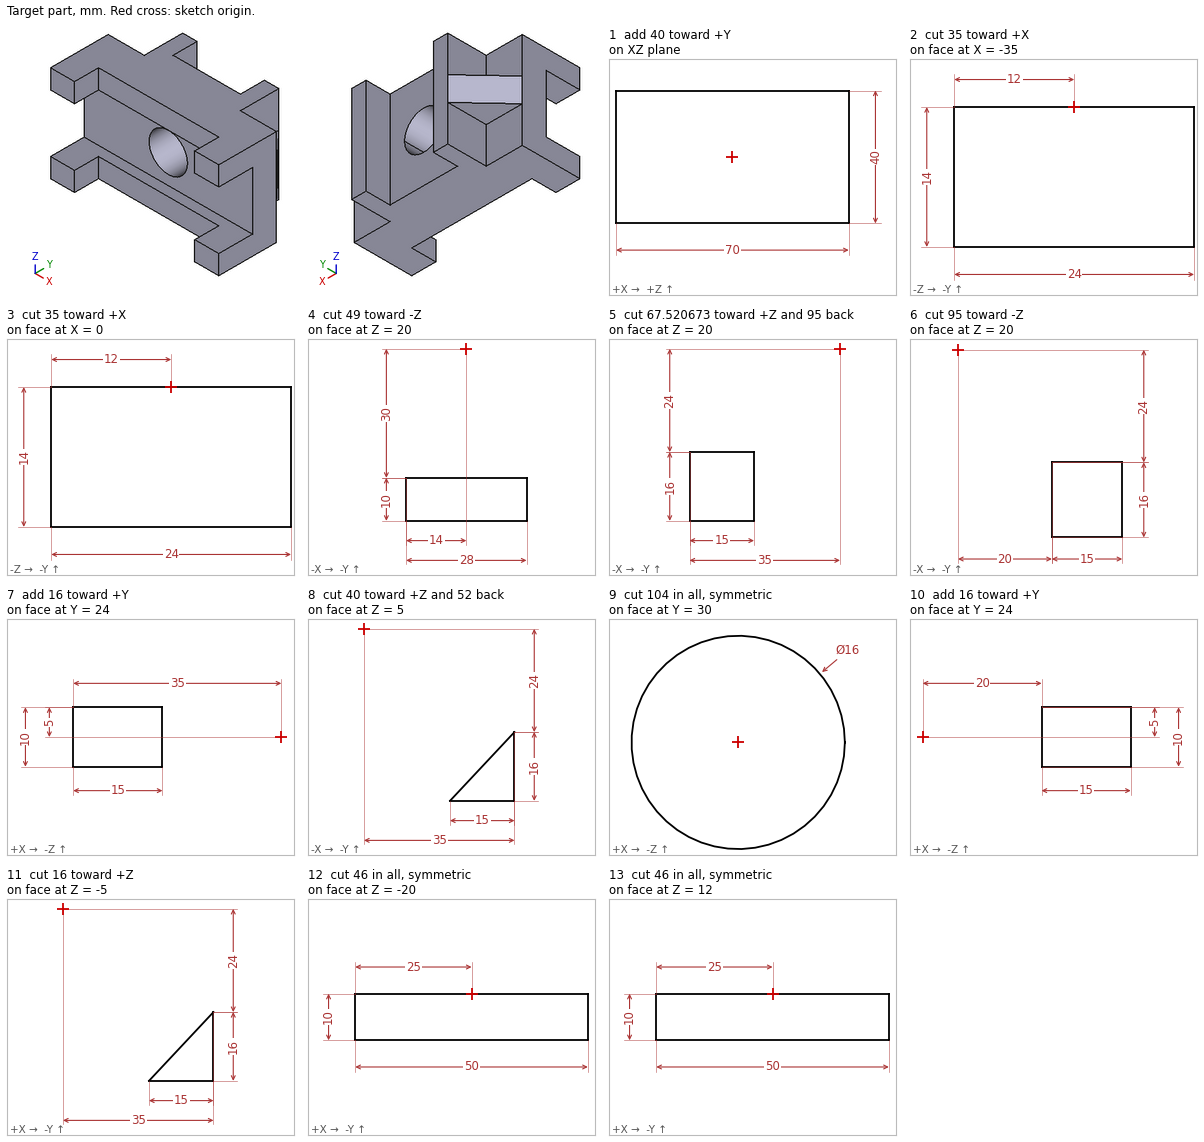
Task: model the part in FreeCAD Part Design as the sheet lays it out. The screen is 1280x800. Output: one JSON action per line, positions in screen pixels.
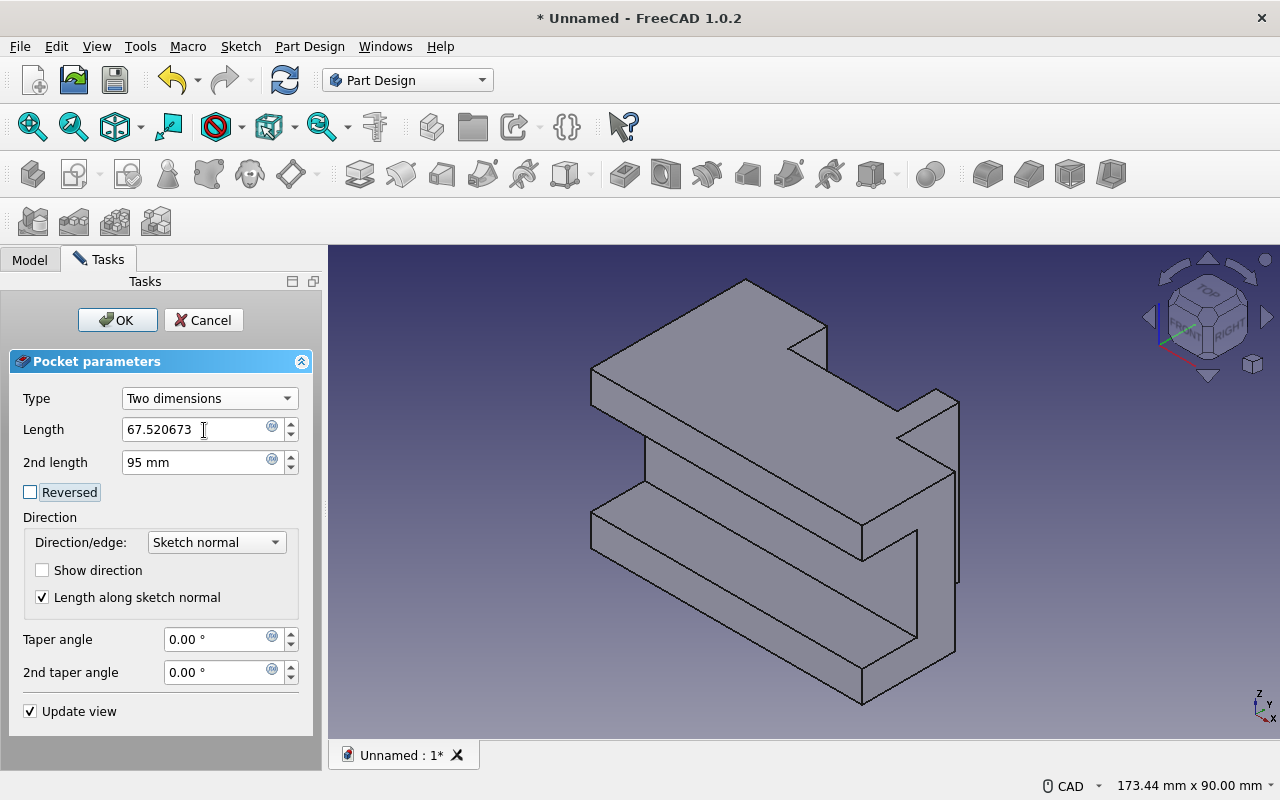
{"action": "left_click", "coordinate": [31, 492]}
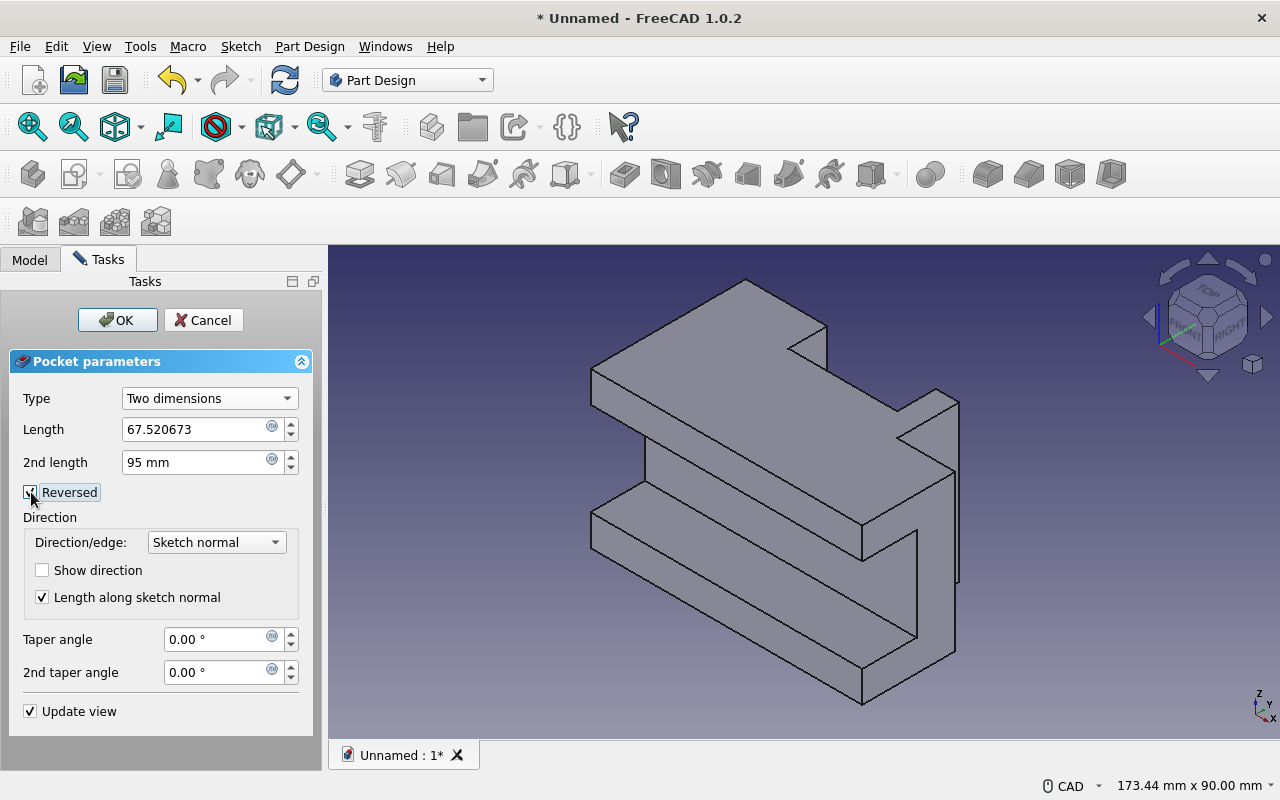
{"action": "left_click", "coordinate": [118, 320]}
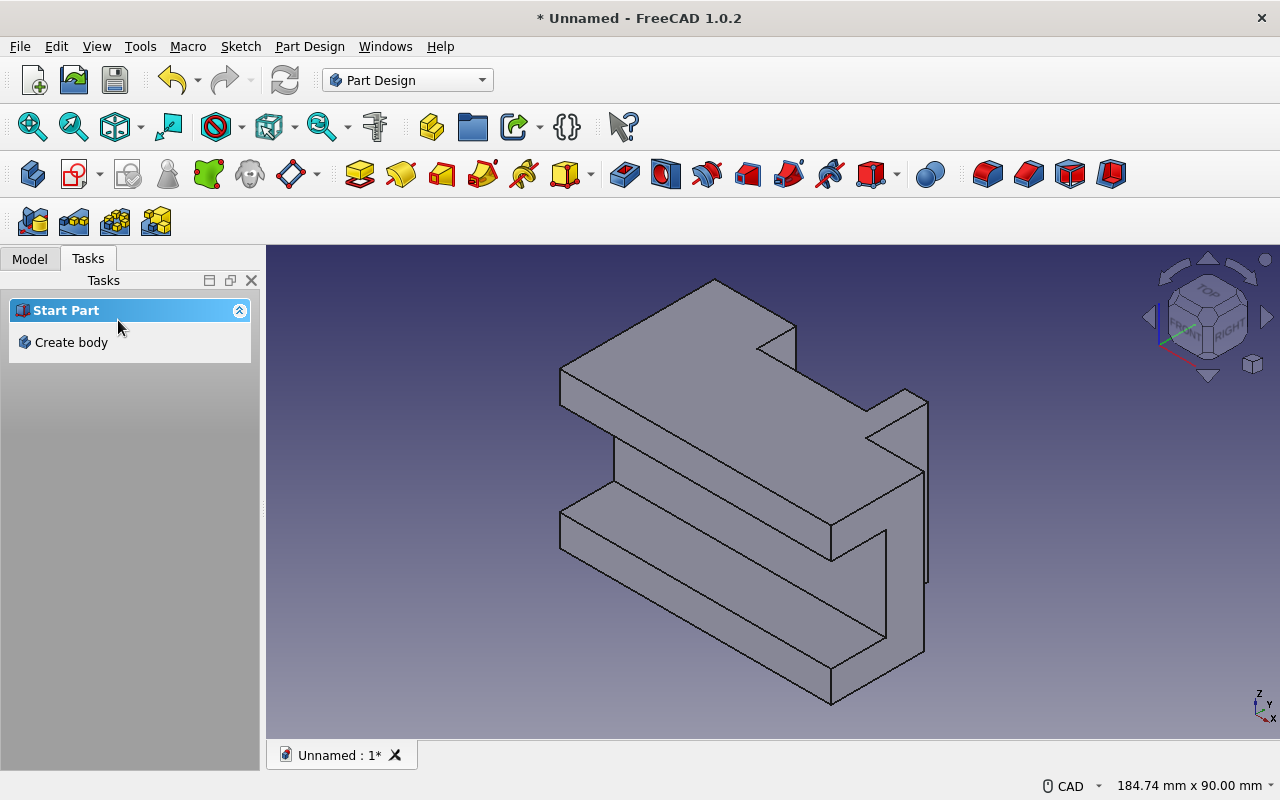
{"action": "left_click", "coordinate": [751, 414]}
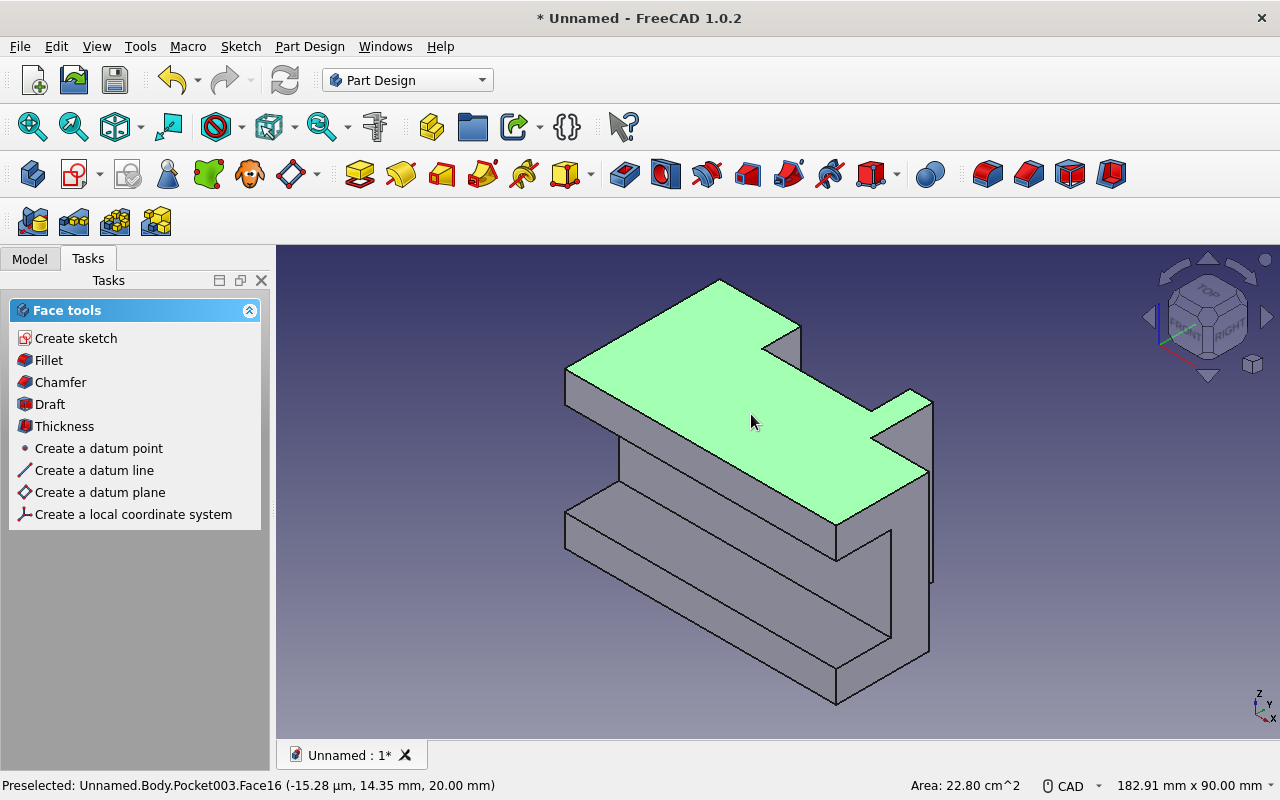
{"action": "left_click", "coordinate": [74, 174]}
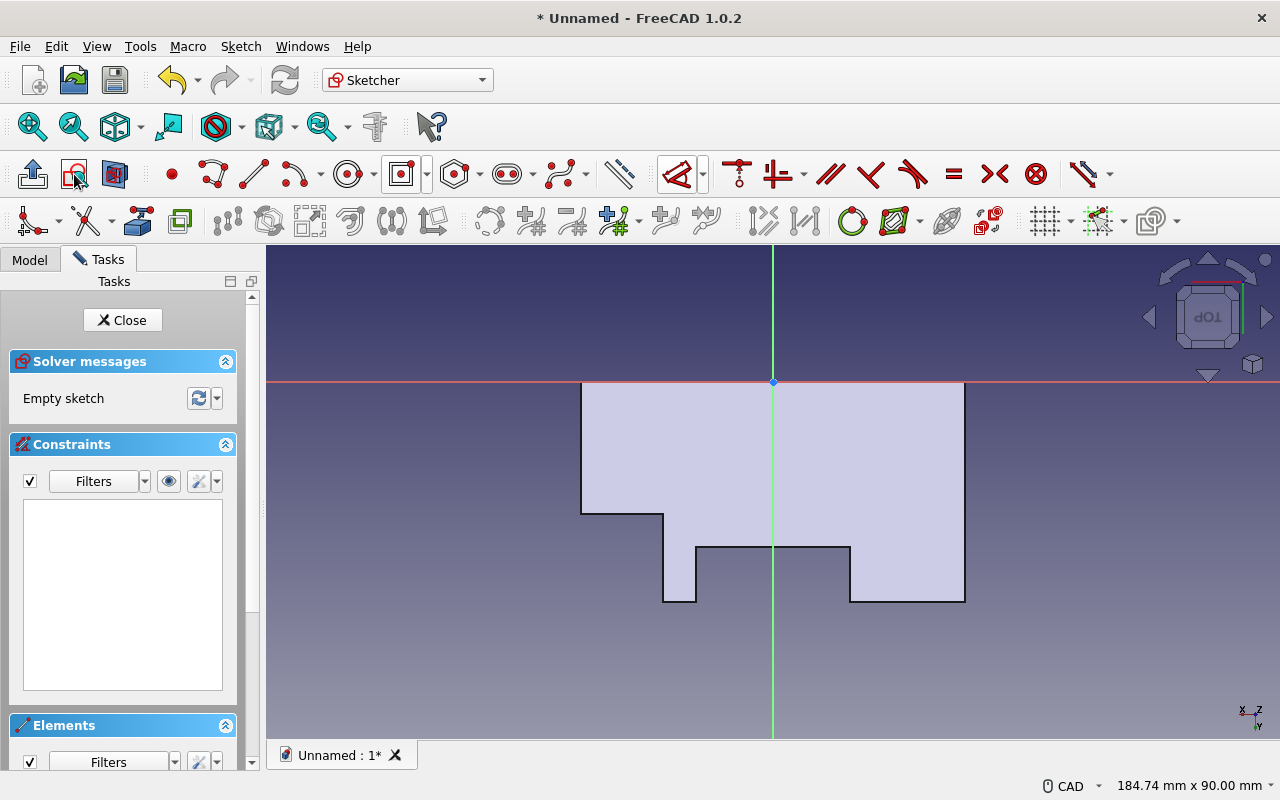
{"action": "scroll", "coordinate": [1019, 586], "scroll_direction": "up", "scroll_amount": 6}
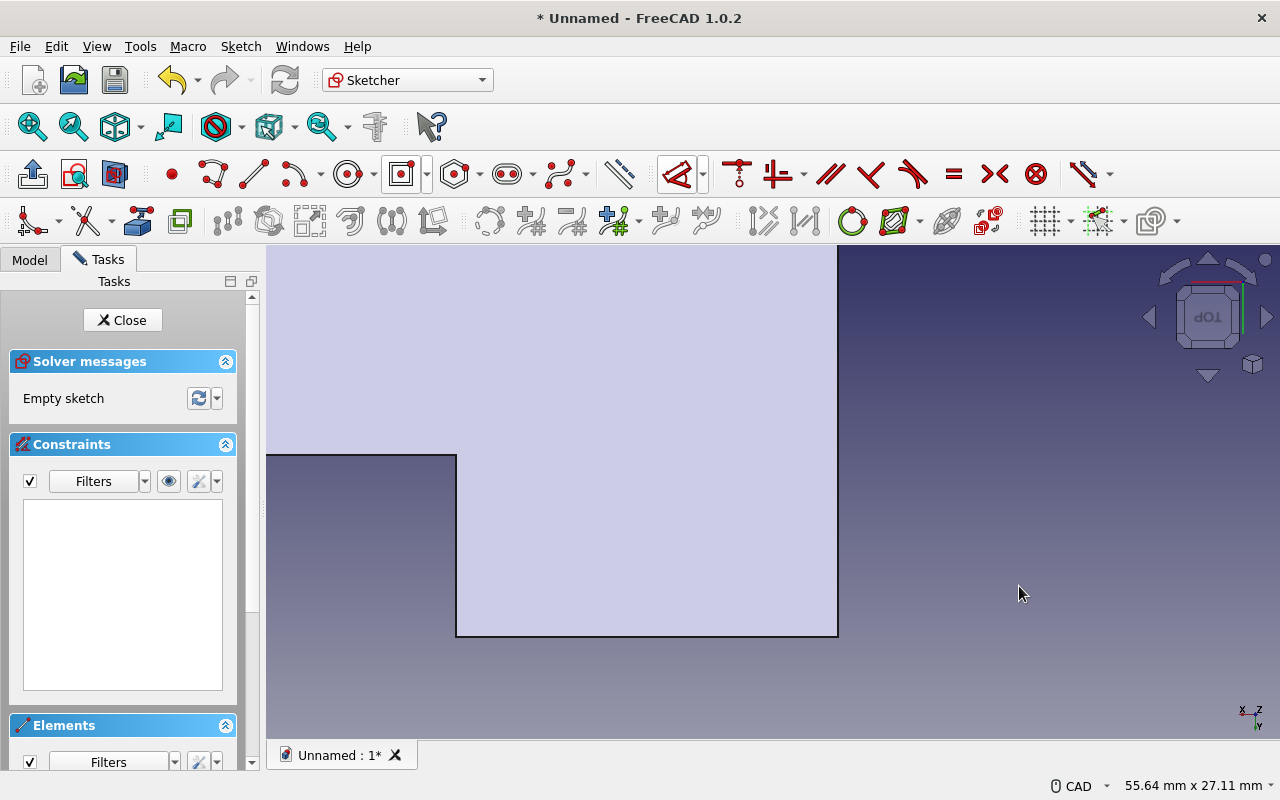
{"action": "key", "text": "g r"}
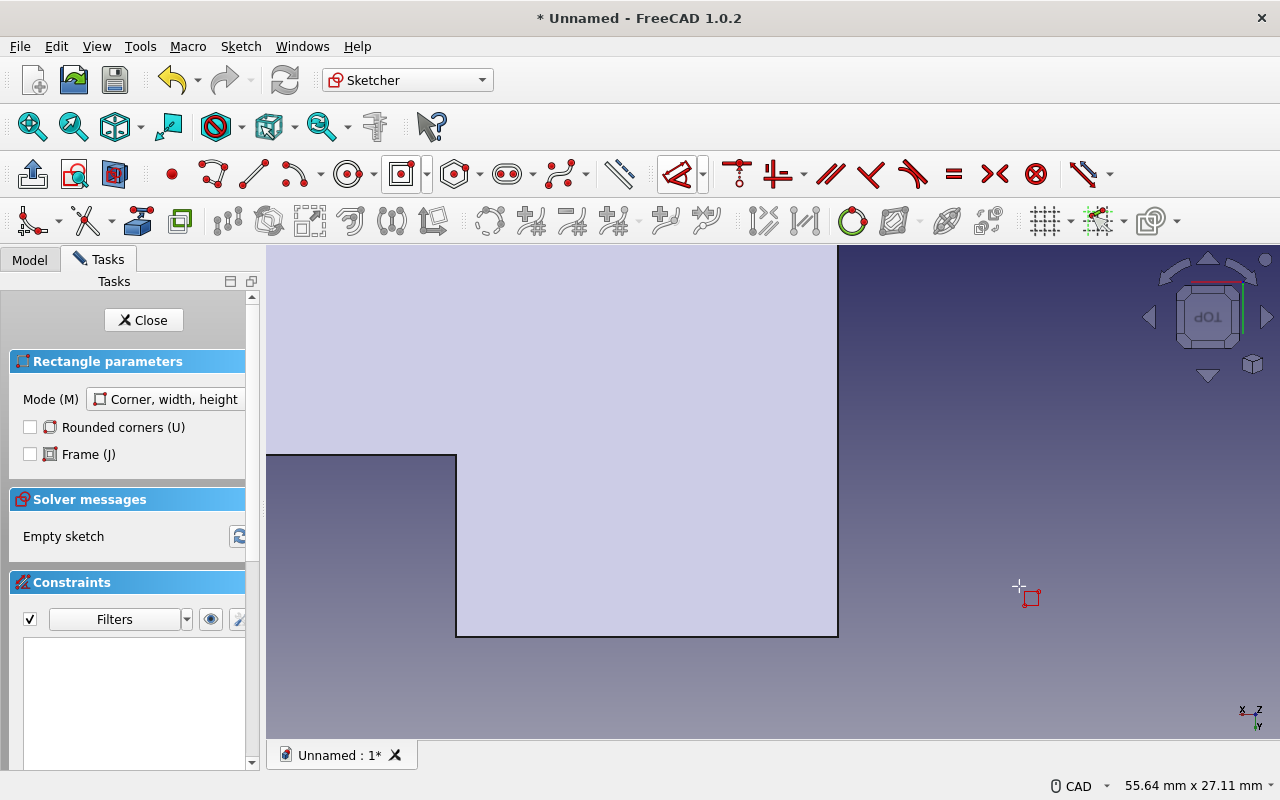
{"action": "left_click", "coordinate": [565, 345]}
{"action": "left_click", "coordinate": [838, 637]}
{"action": "key", "text": "Escape"}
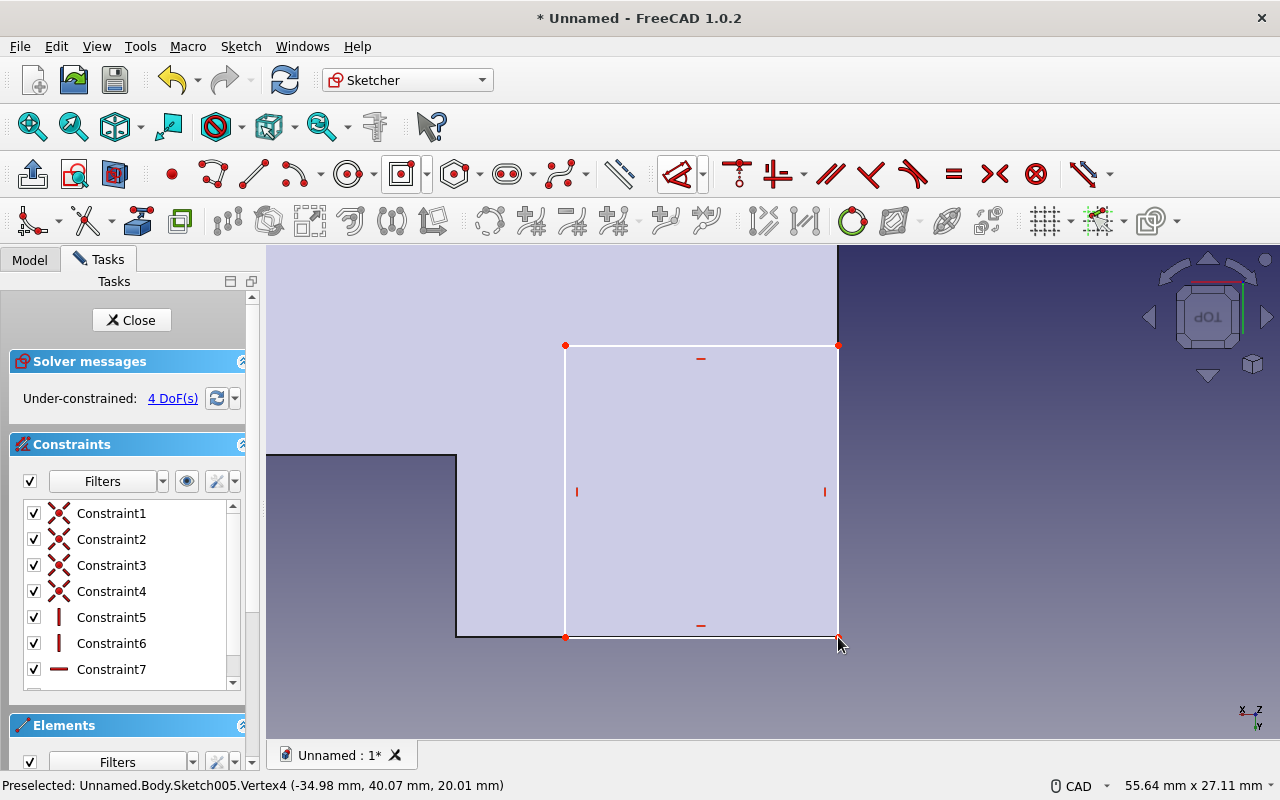
{"action": "left_click", "coordinate": [565, 434]}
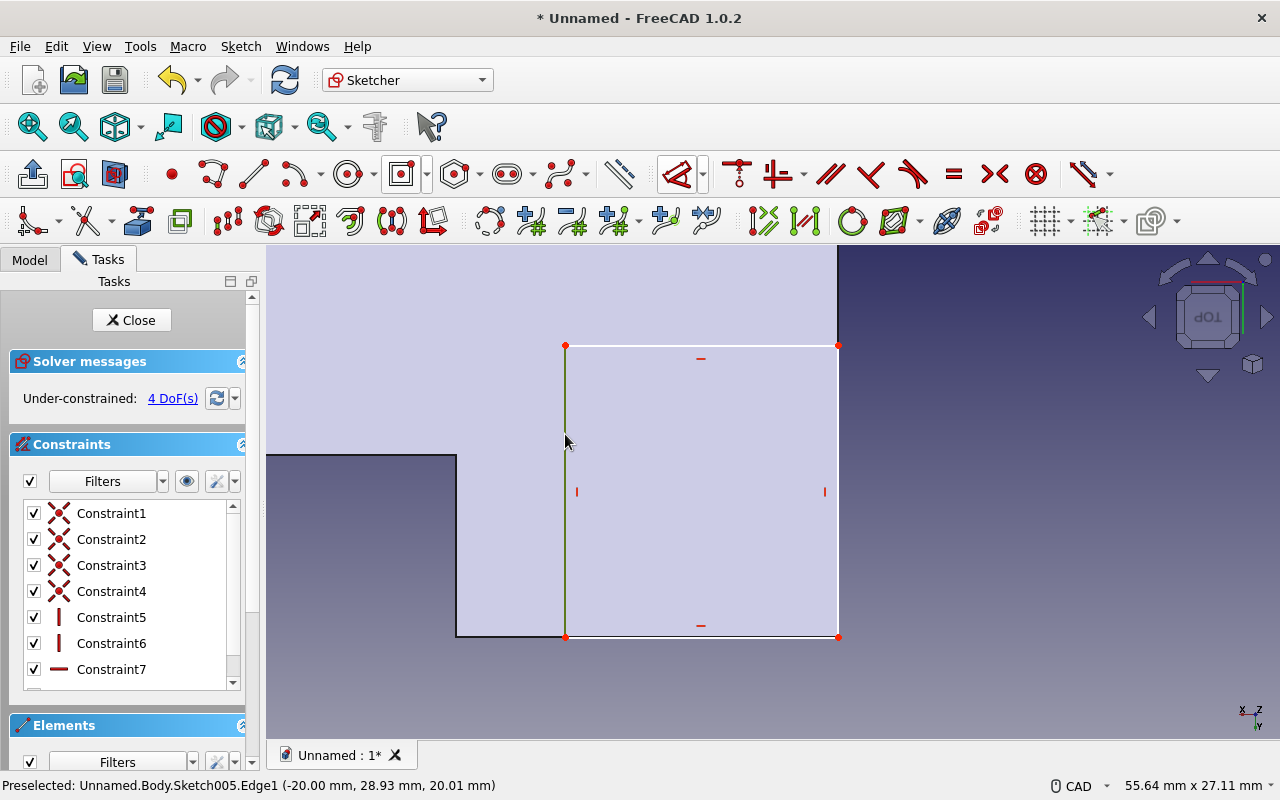
{"action": "key", "text": "i"}